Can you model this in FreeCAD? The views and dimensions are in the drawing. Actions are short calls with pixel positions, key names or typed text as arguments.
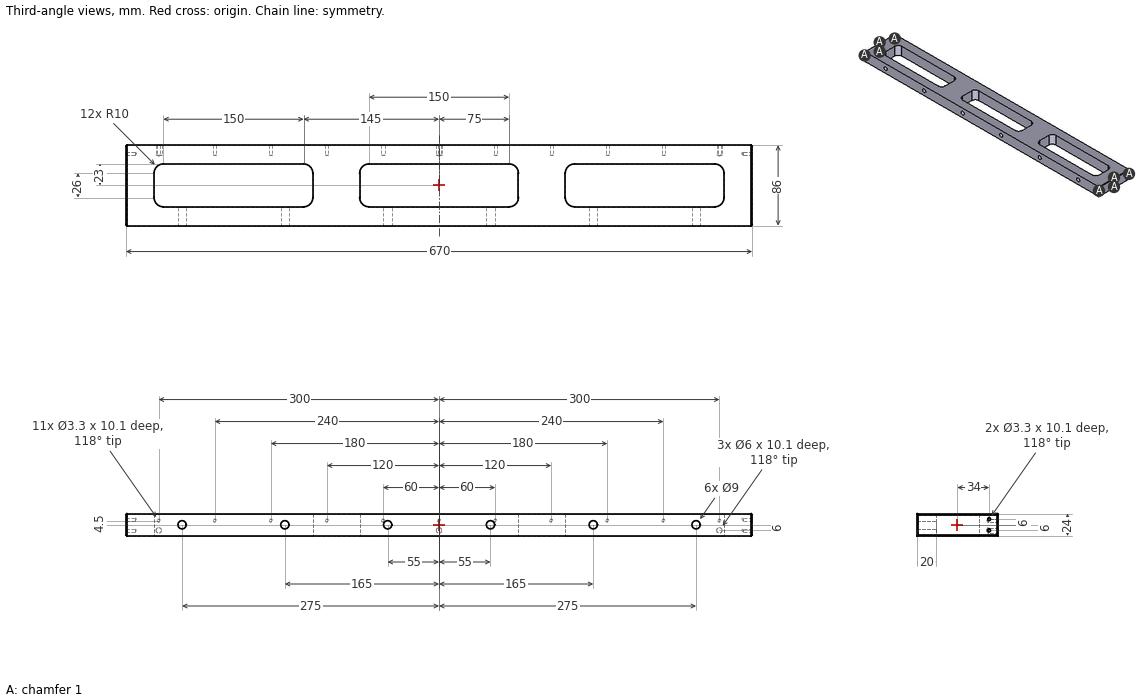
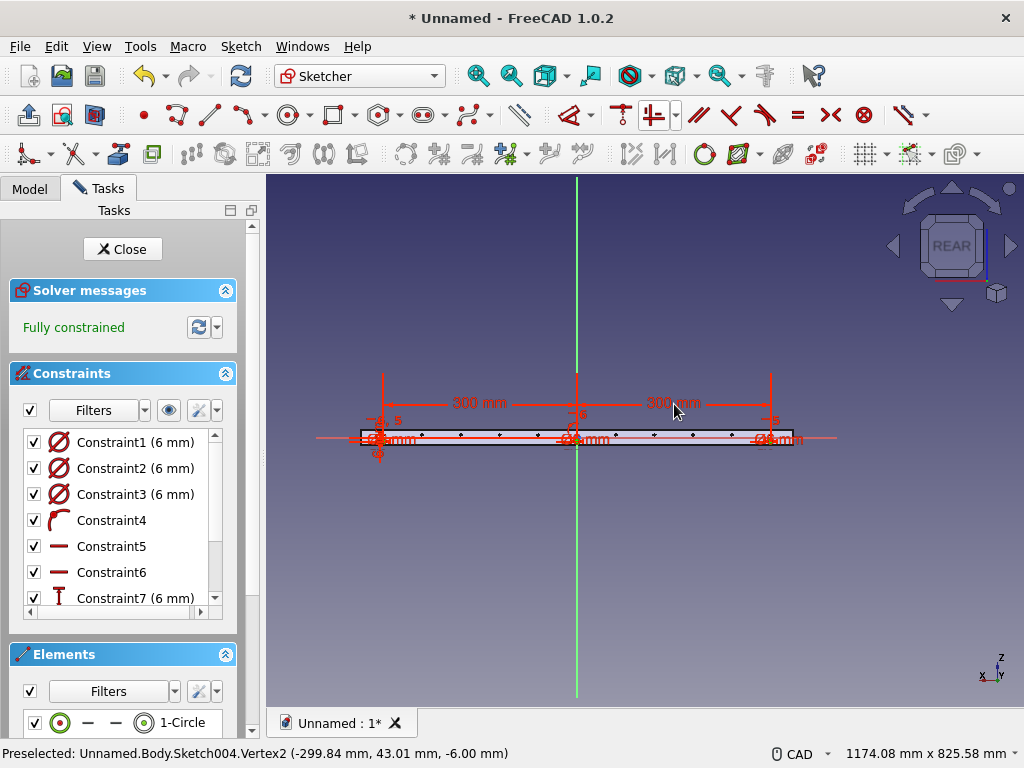
click(123, 249)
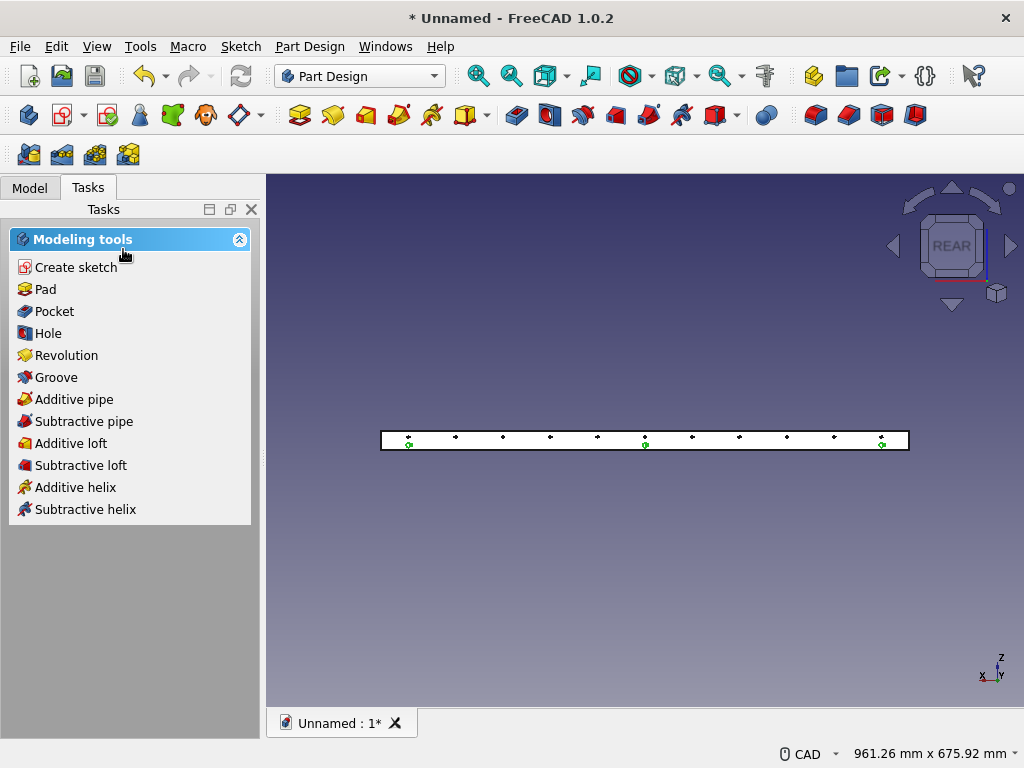
click(550, 116)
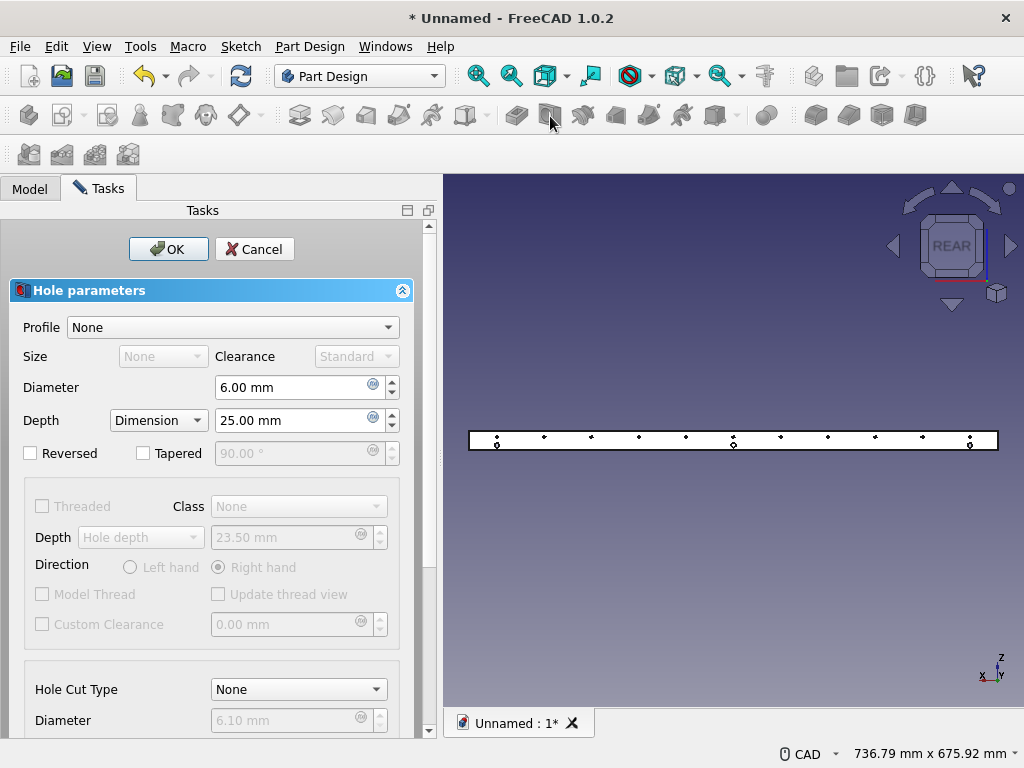
triple_click(300, 388)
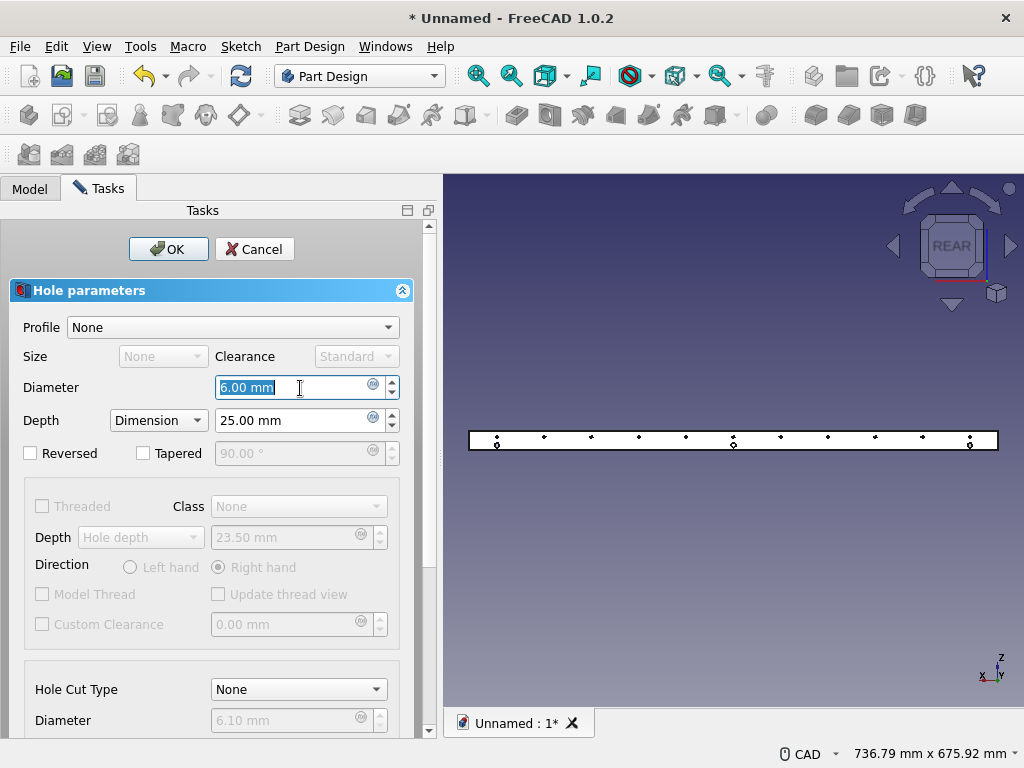
text(6)
key(Tab)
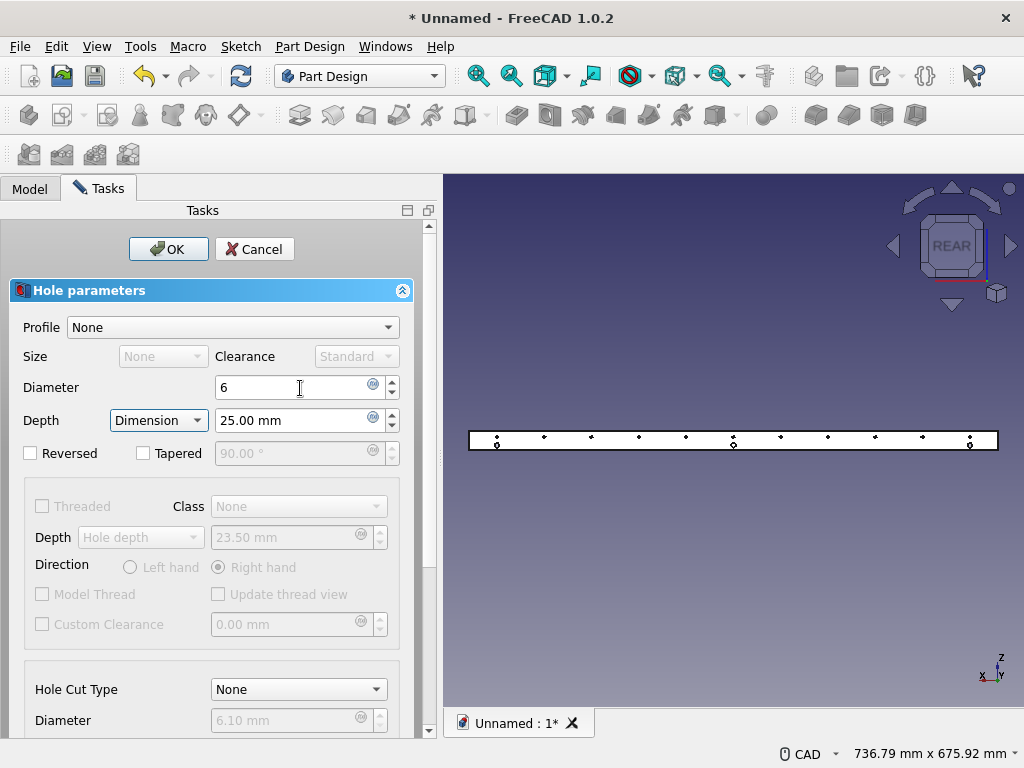
triple_click(300, 420)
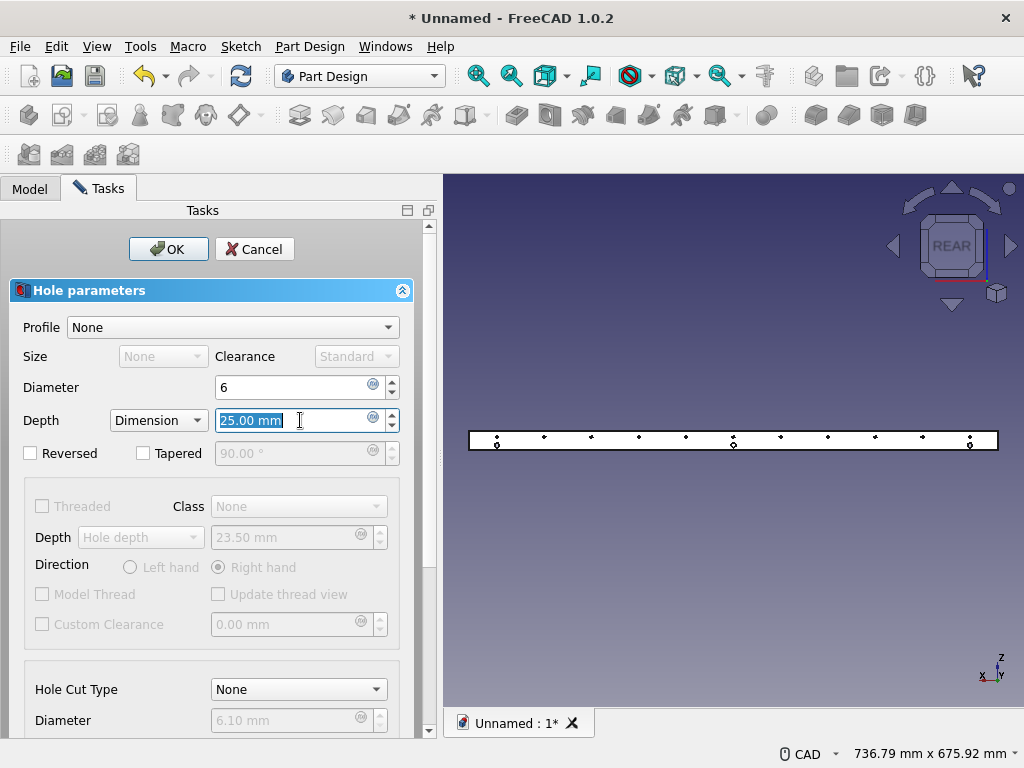
text(10.1)
key(Tab)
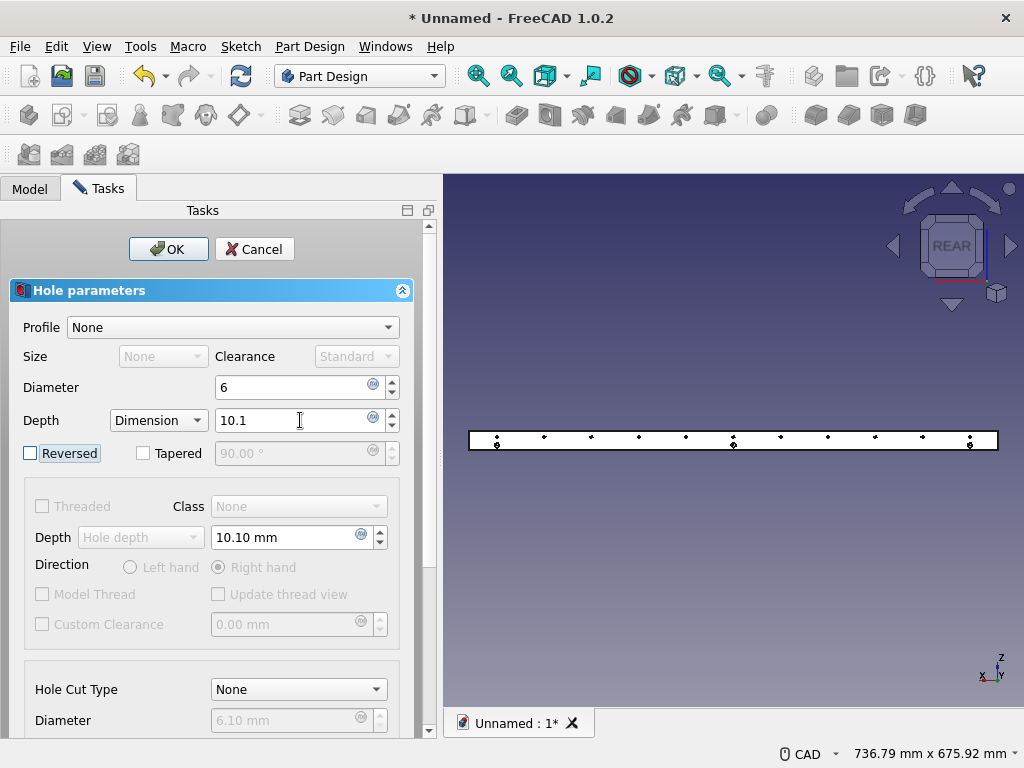
click(169, 249)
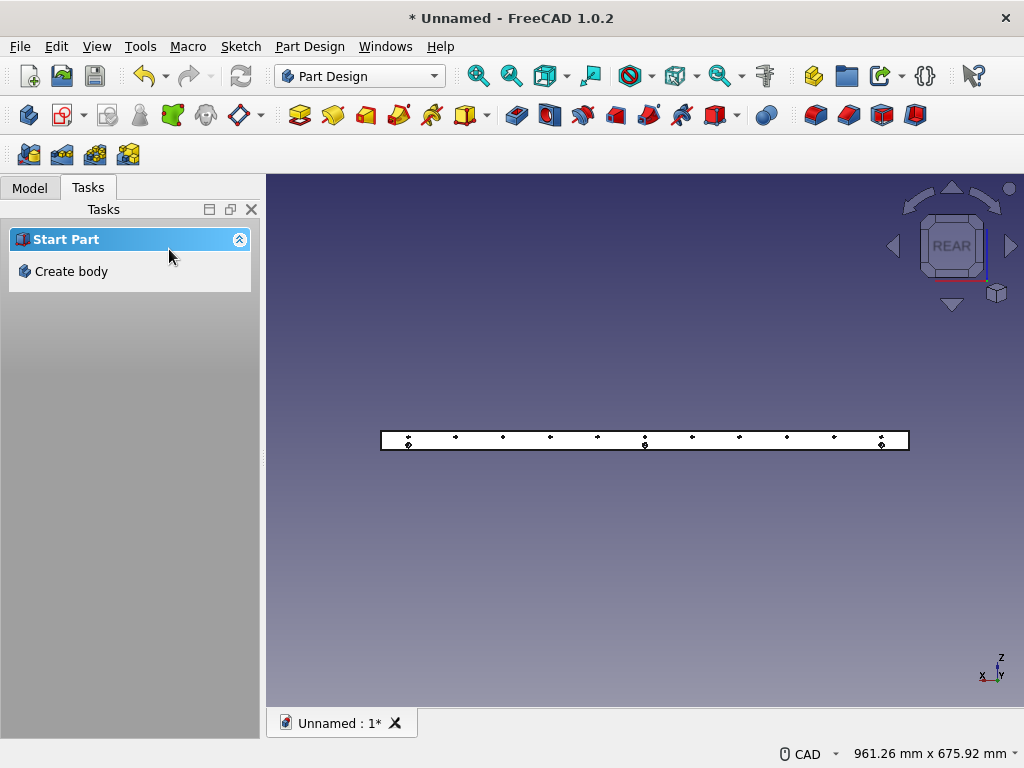
key(0)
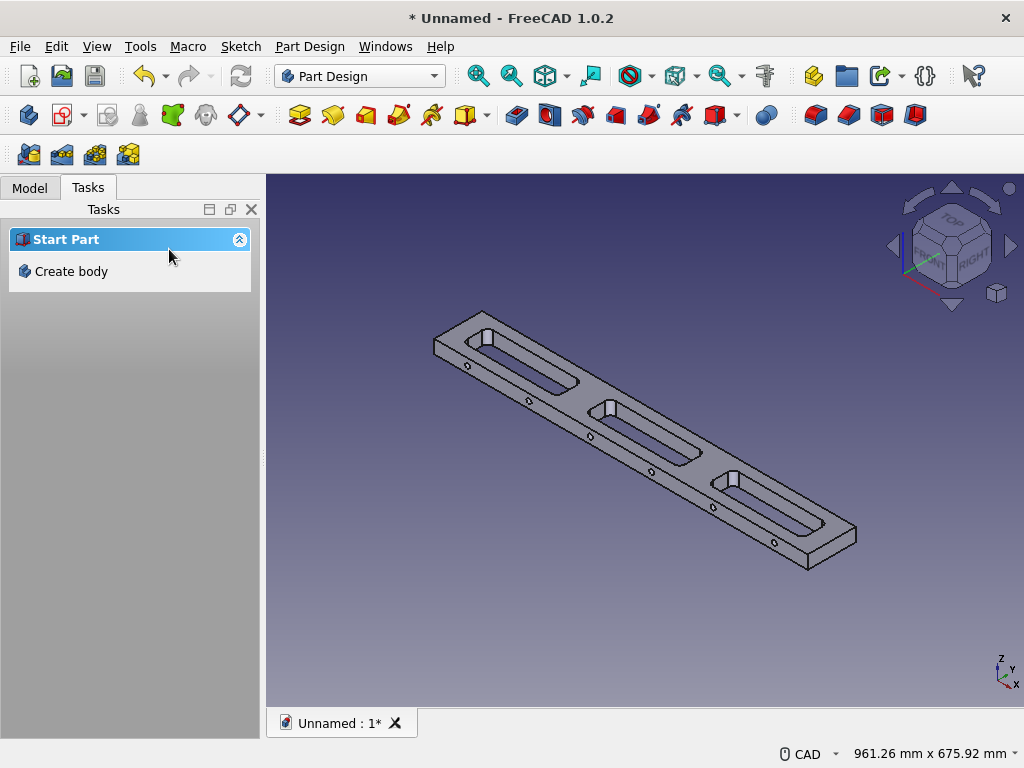
key(2)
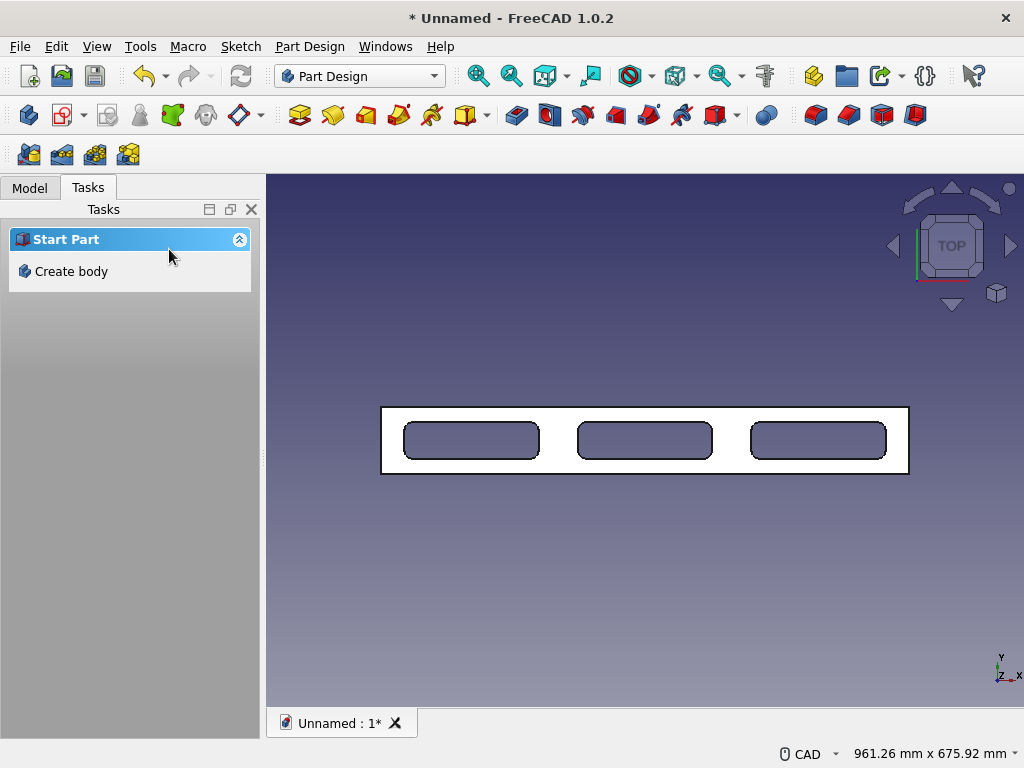
key(1)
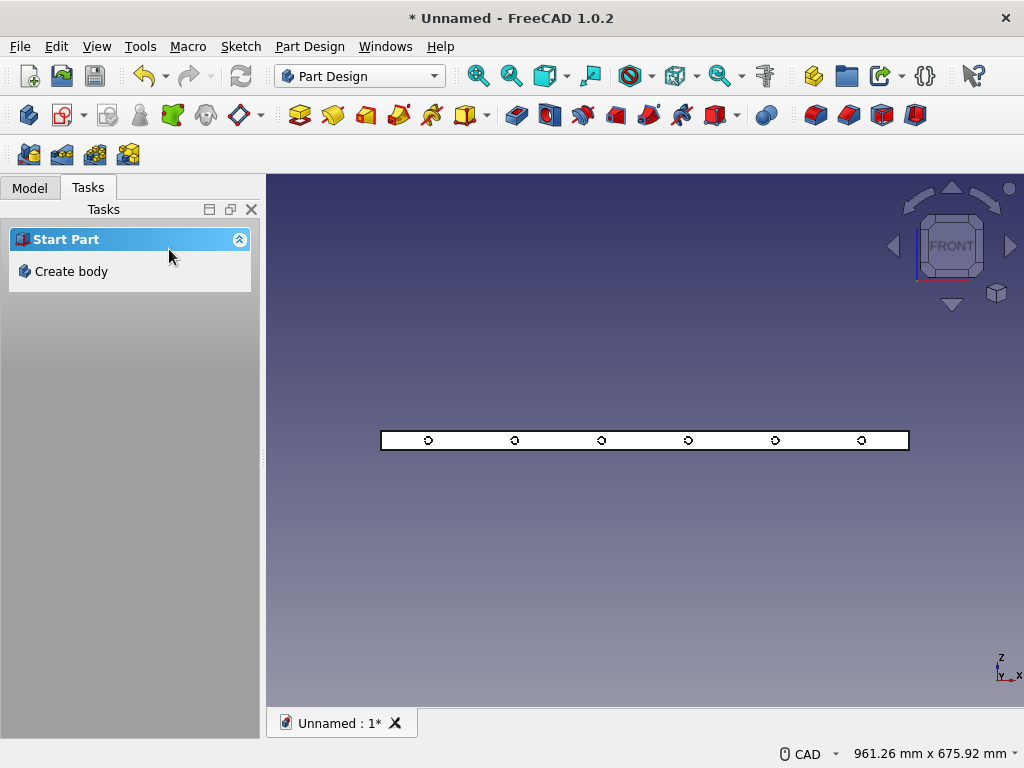
key(3)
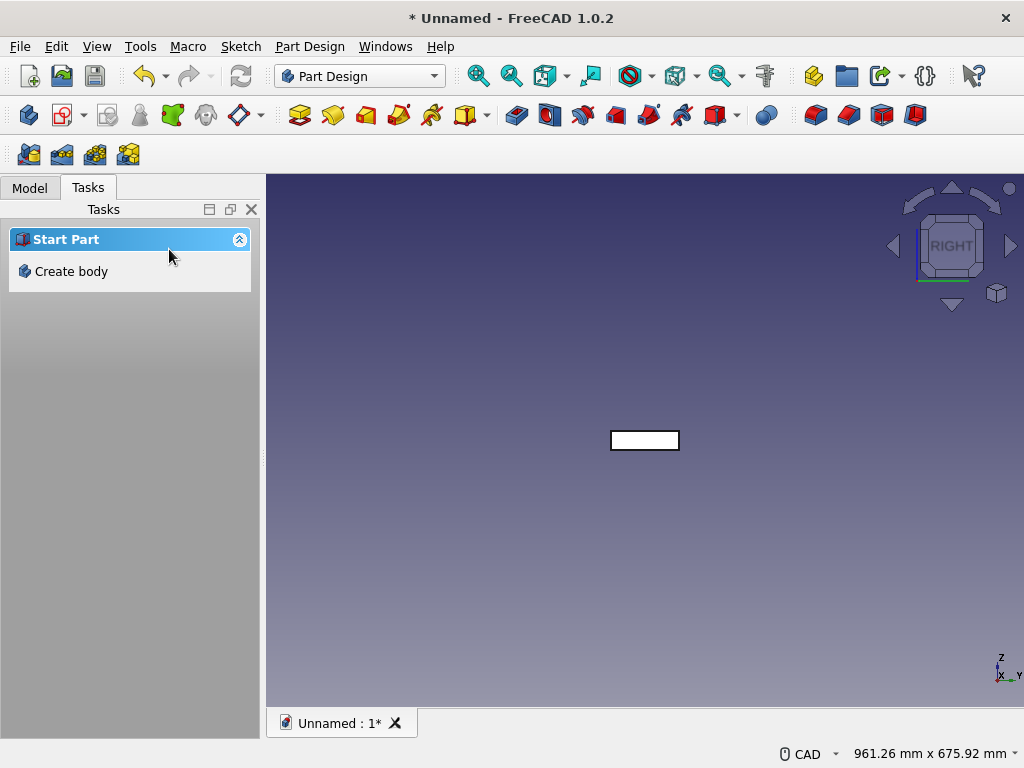
key(v)
key(f)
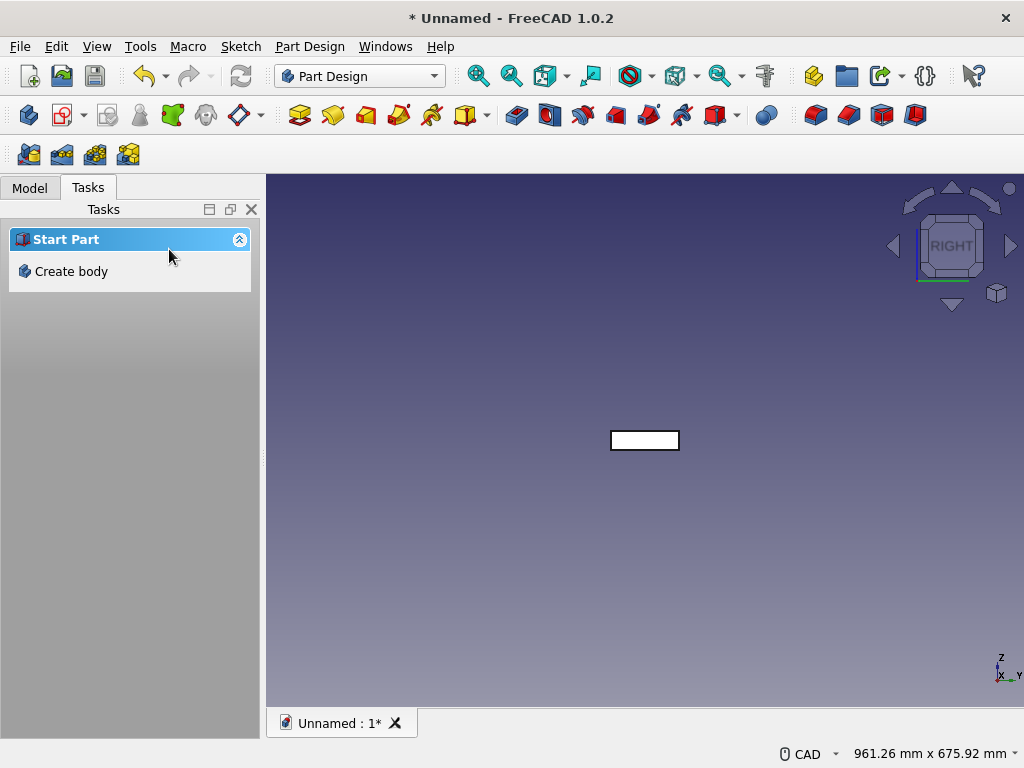
click(664, 439)